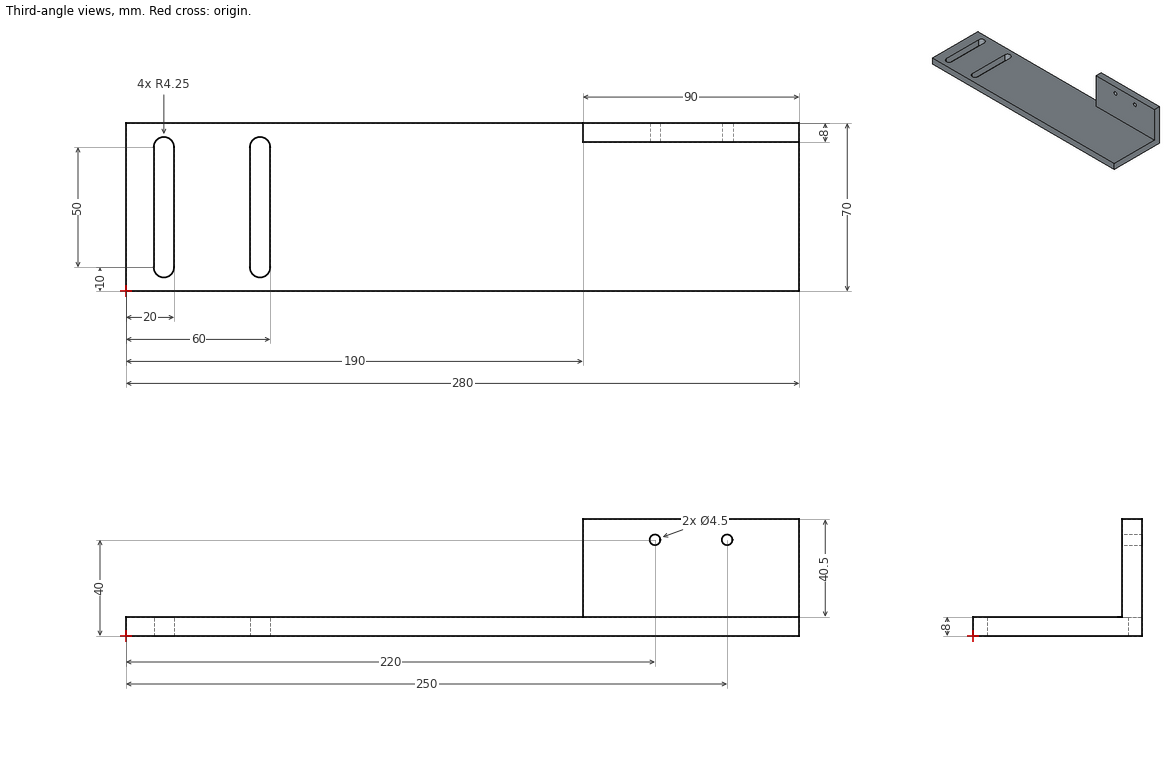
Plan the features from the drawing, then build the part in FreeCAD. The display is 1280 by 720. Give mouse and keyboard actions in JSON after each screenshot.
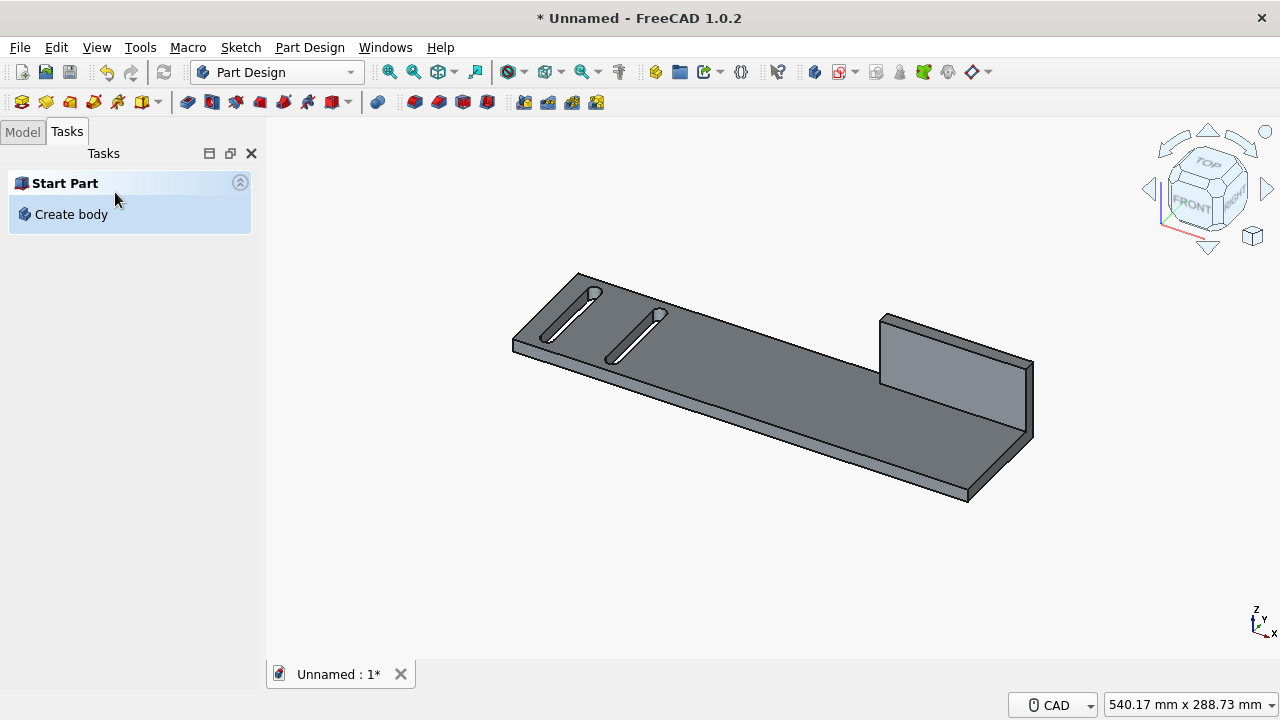
{"action": "key", "text": "4"}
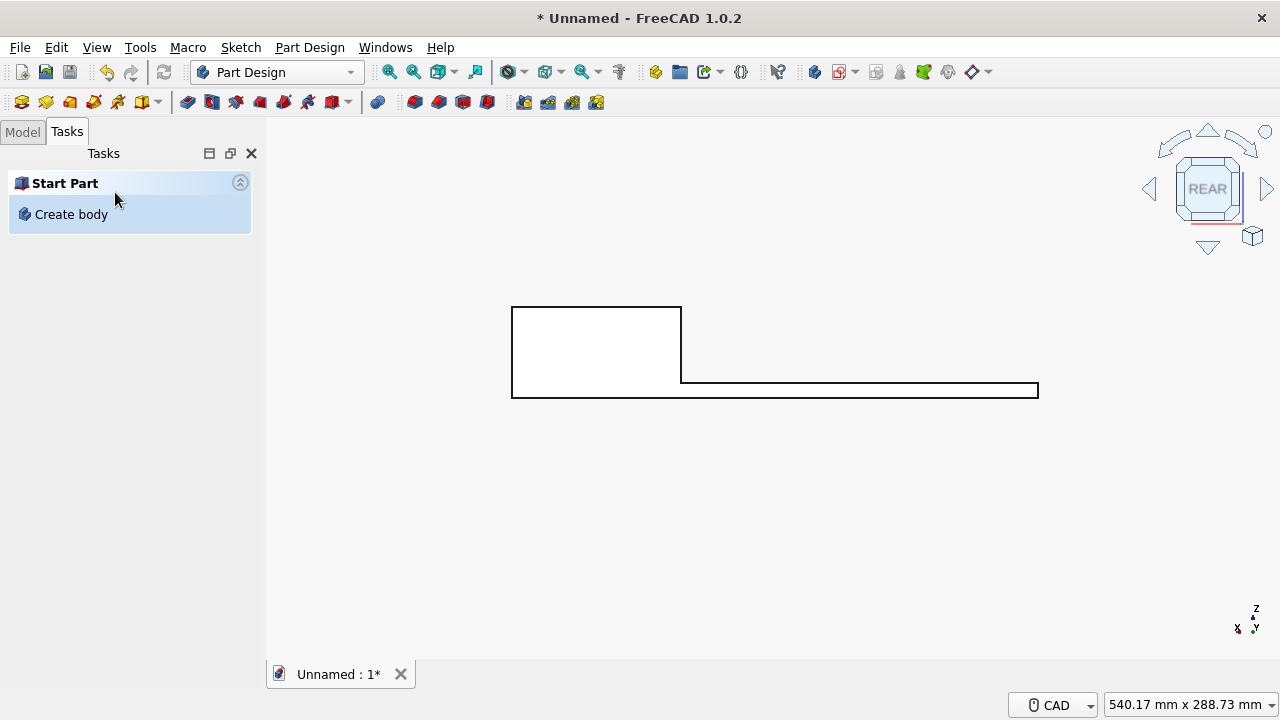
{"action": "left_click", "coordinate": [625, 352]}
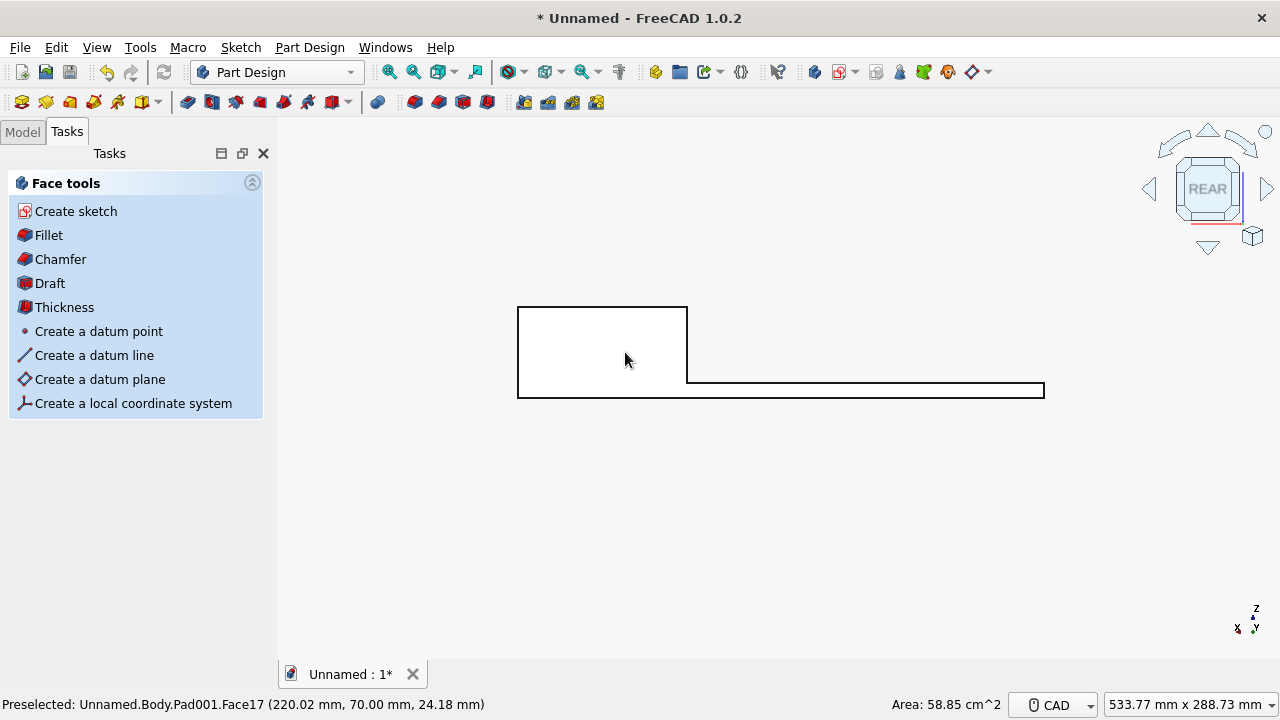
{"action": "left_click", "coordinate": [840, 72]}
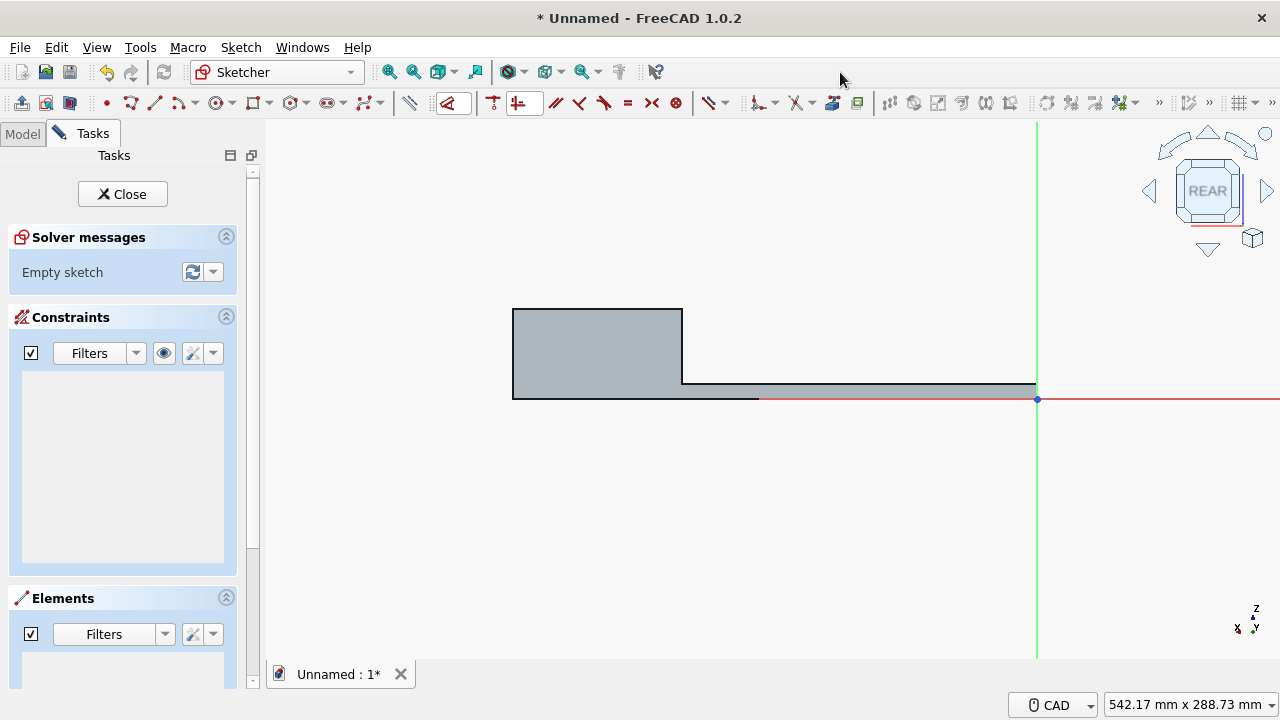
{"action": "scroll", "coordinate": [584, 317], "scroll_direction": "up", "scroll_amount": 11}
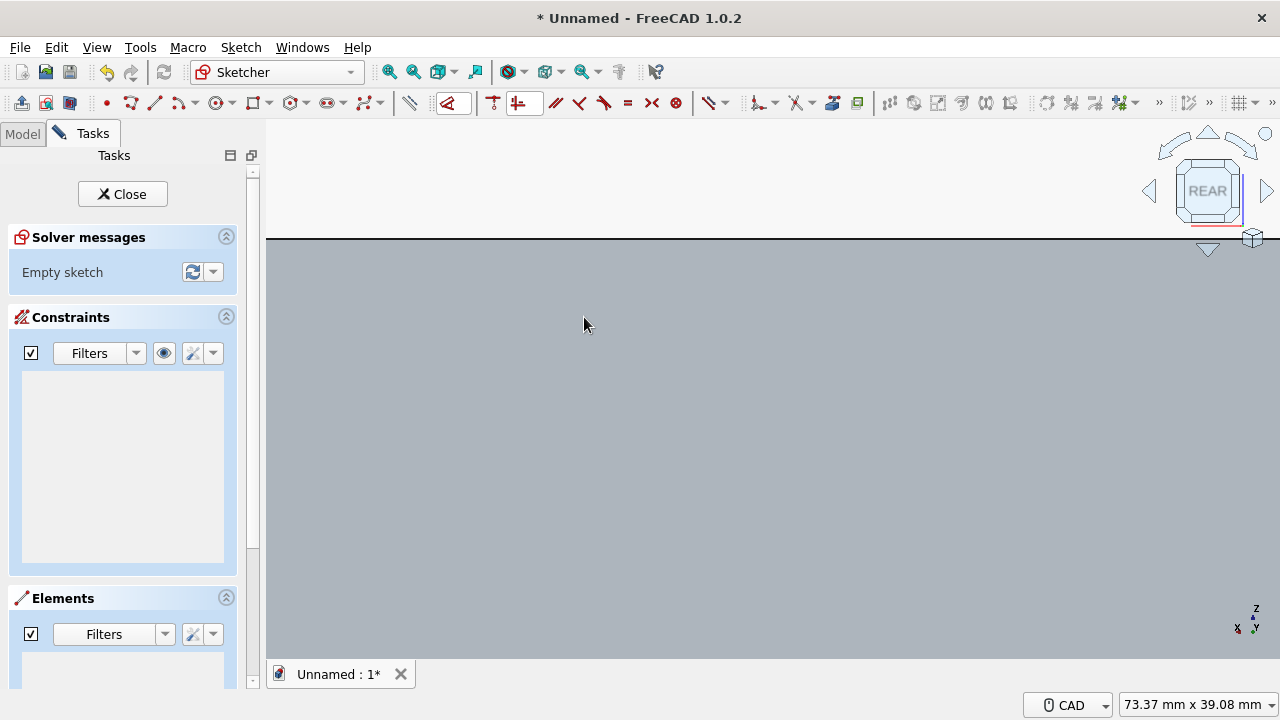
{"action": "key", "text": "g c"}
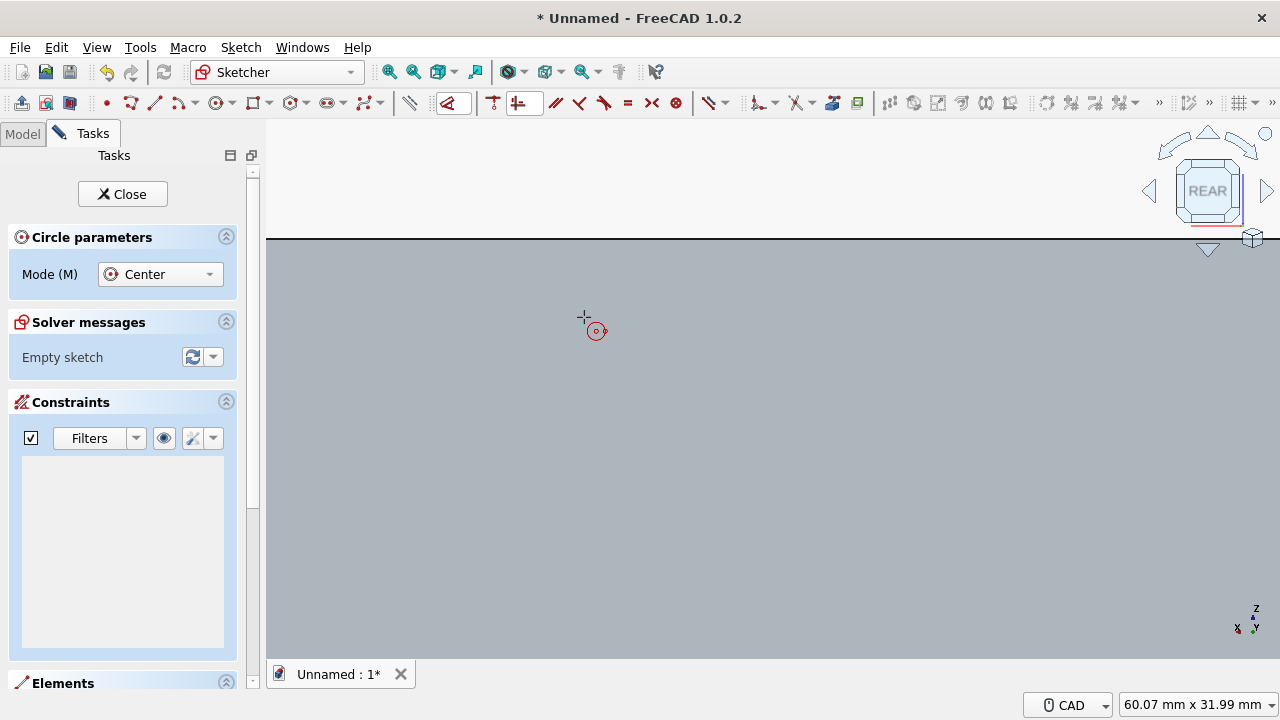
{"action": "left_click", "coordinate": [957, 382]}
{"action": "mouse_move", "coordinate": [984, 355]}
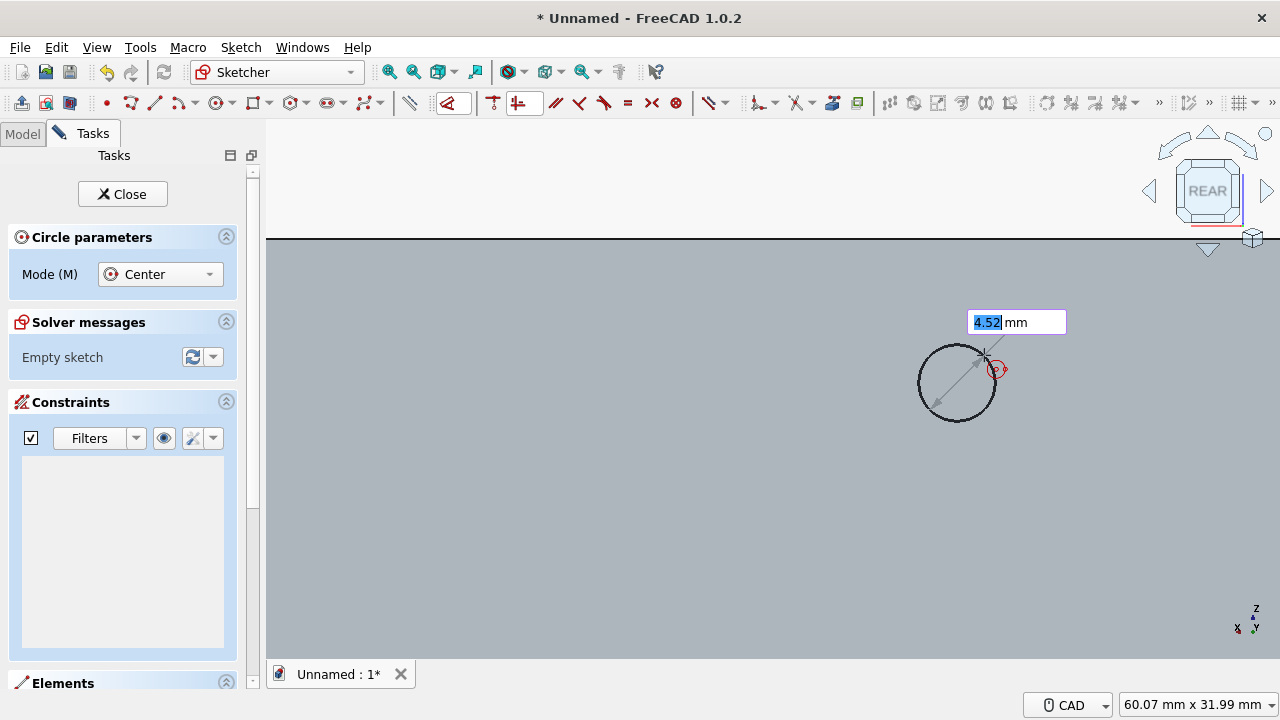
{"action": "type", "text": "4.5"}
{"action": "key", "text": "Return"}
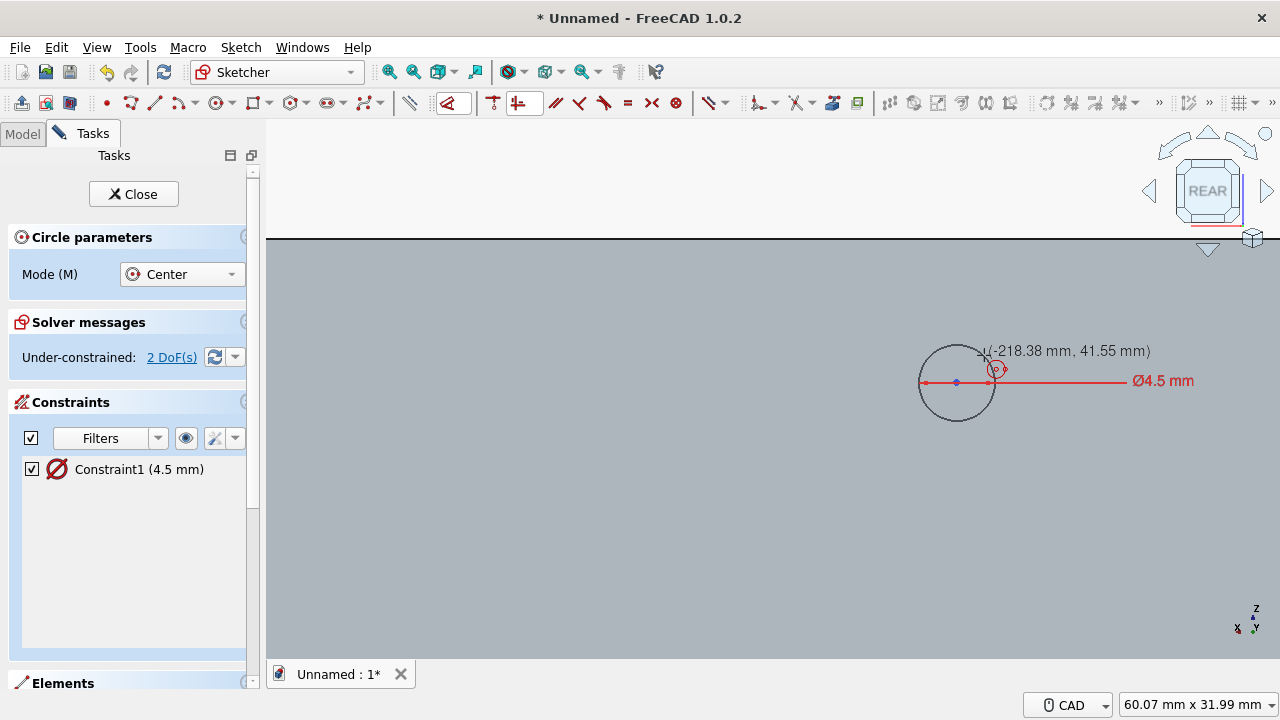
{"action": "left_click", "coordinate": [450, 382]}
{"action": "mouse_move", "coordinate": [477, 355]}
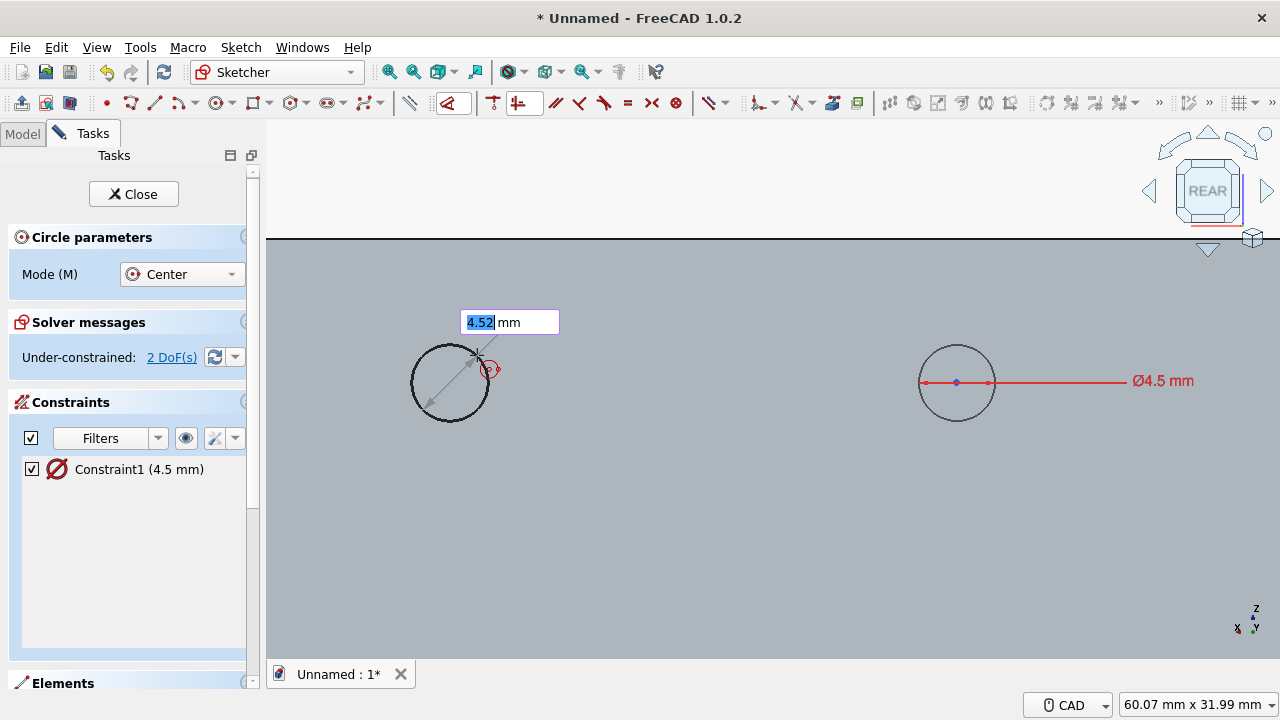
{"action": "type", "text": "4.5"}
{"action": "key", "text": "Return"}
{"action": "key", "text": "Escape"}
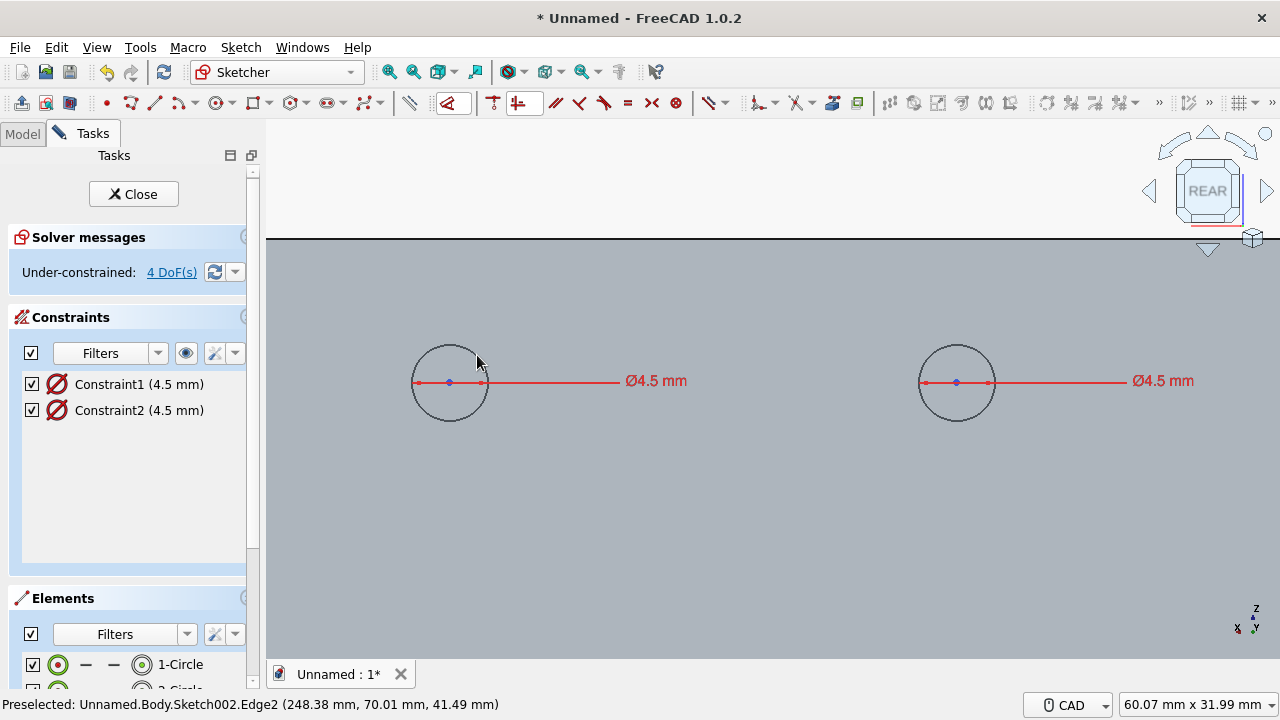
{"action": "left_click", "coordinate": [957, 383]}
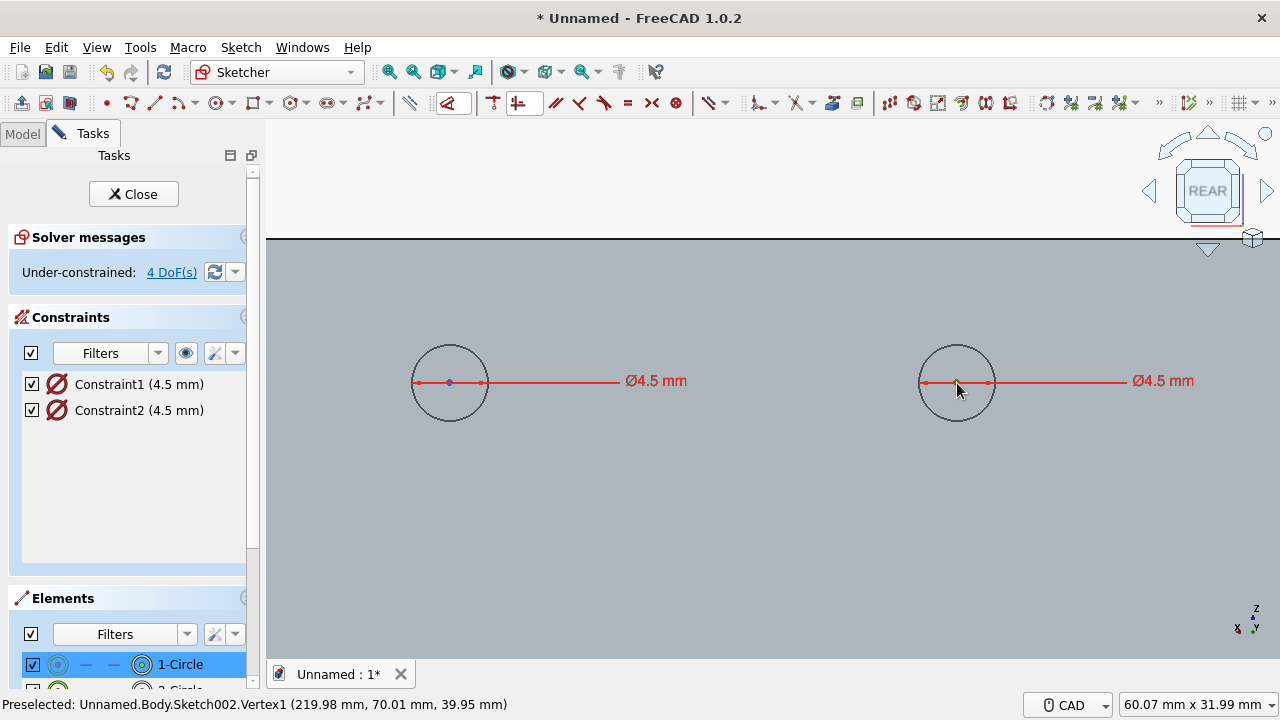
{"action": "left_click", "coordinate": [450, 383]}